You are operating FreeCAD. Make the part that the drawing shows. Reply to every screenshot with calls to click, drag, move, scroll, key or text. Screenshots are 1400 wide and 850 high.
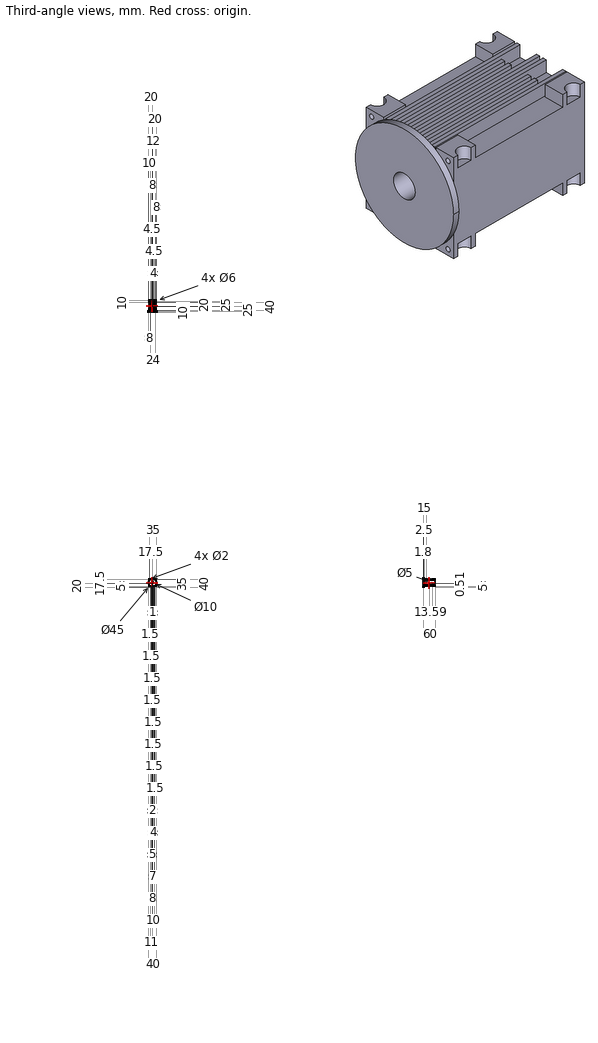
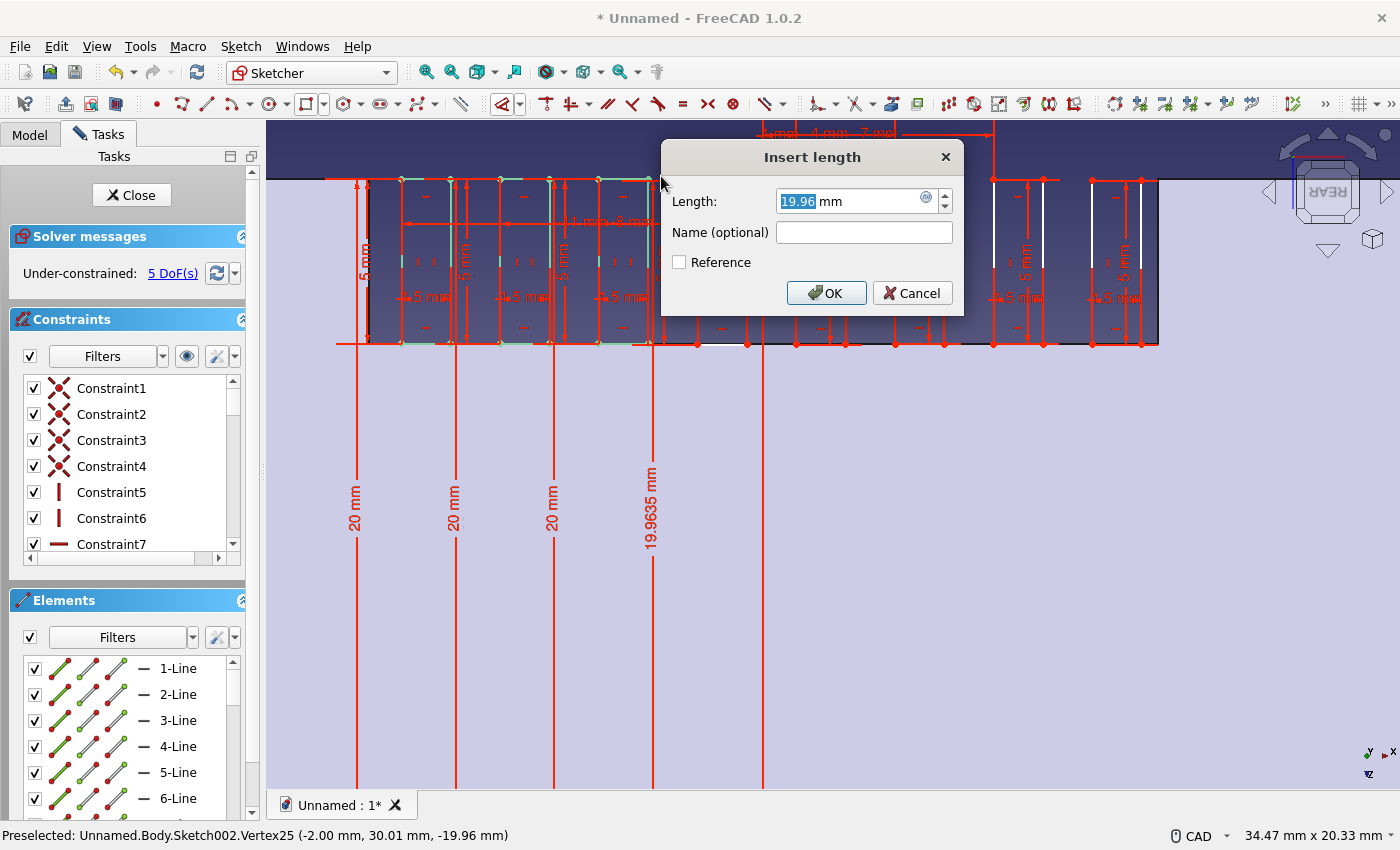
text(20)
key(Return)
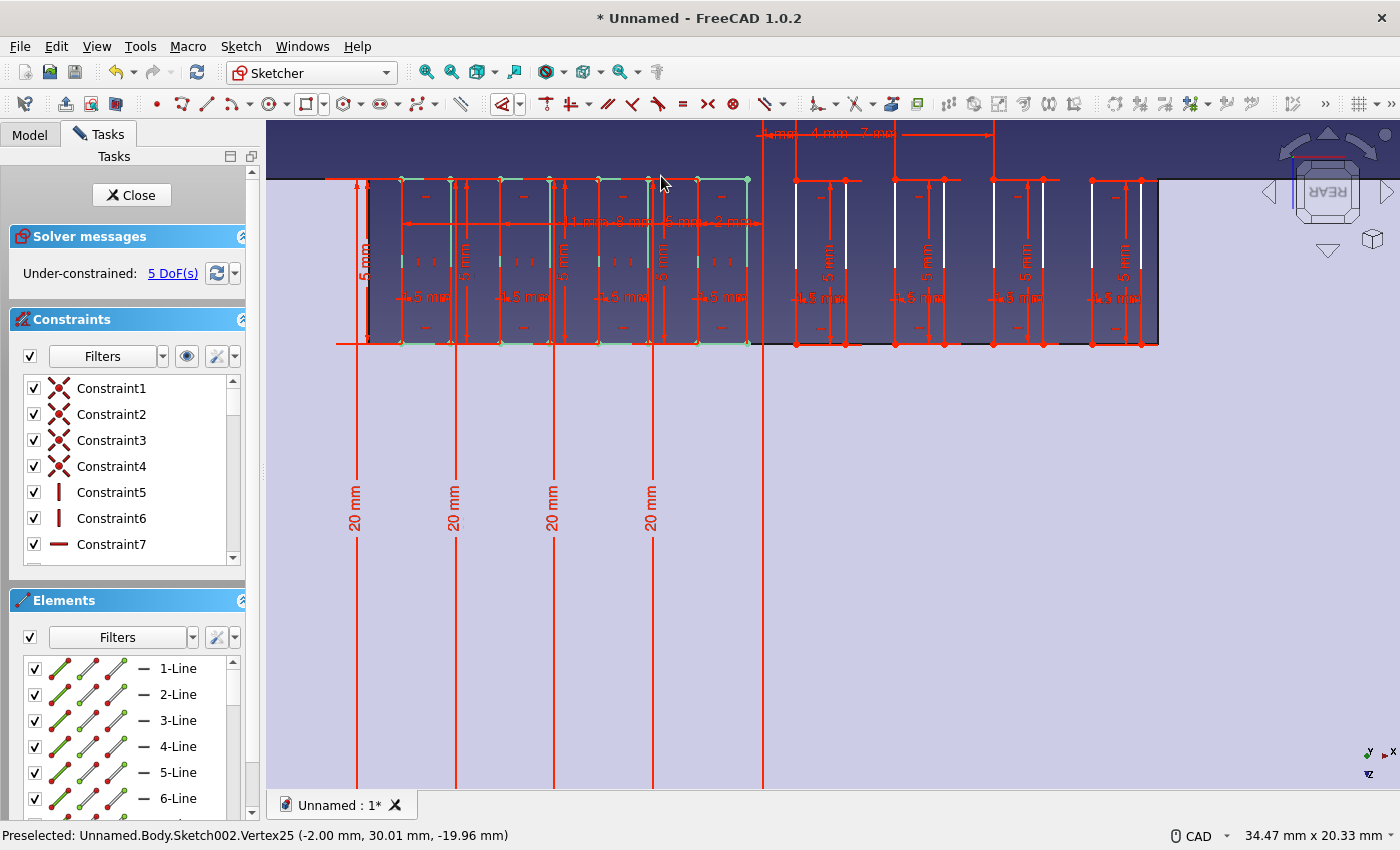
click(796, 181)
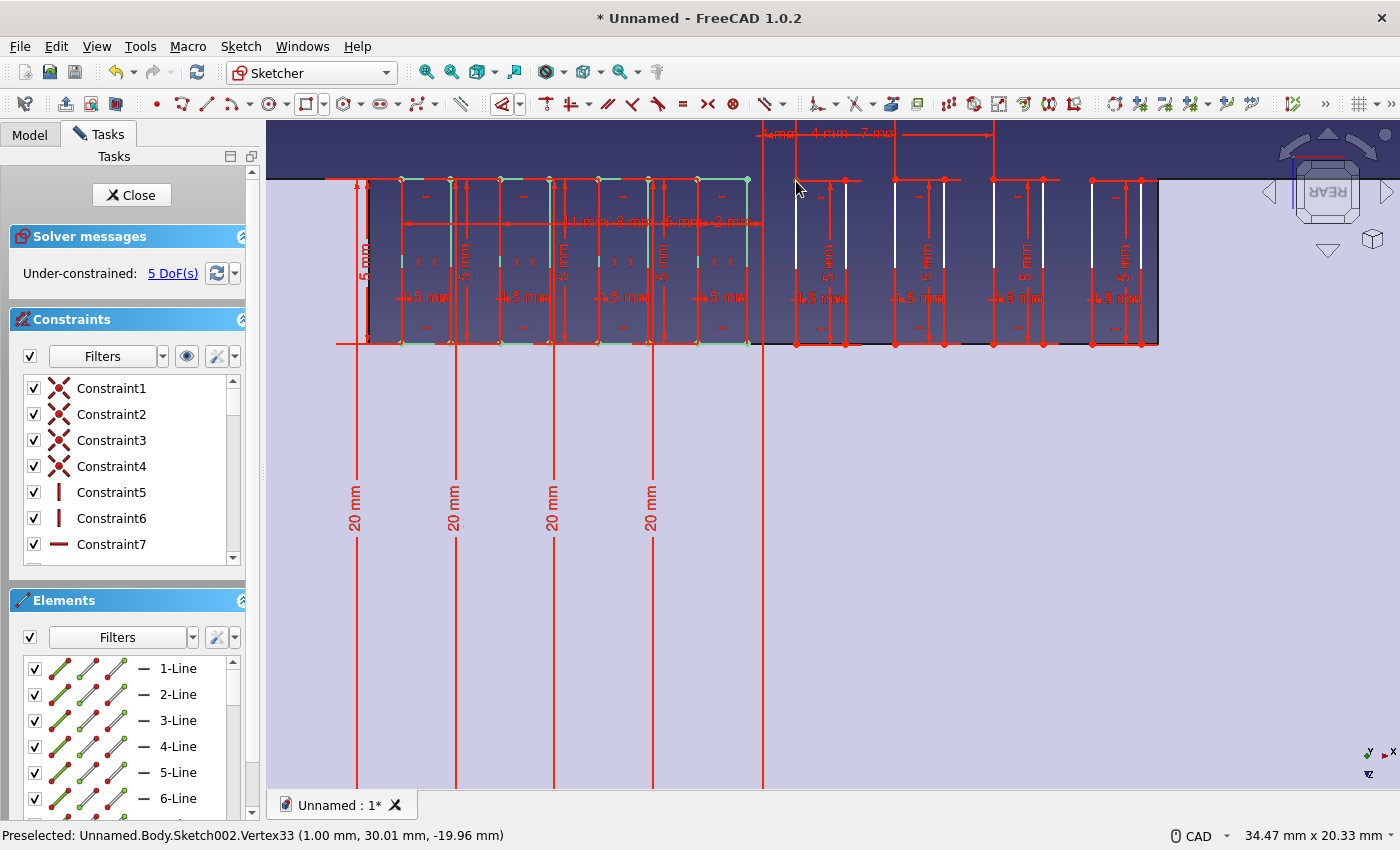
key(i)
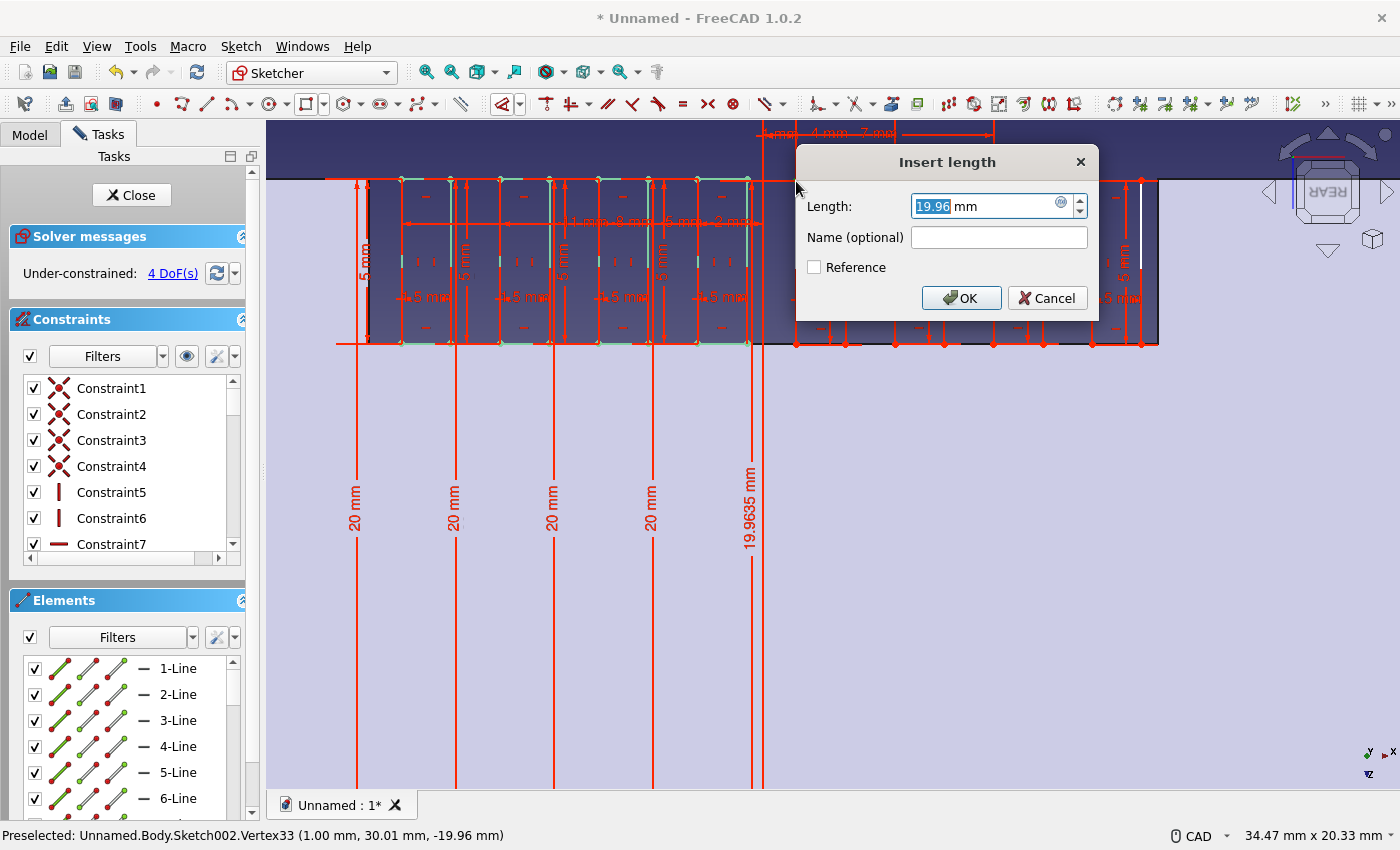
text(20)
key(Return)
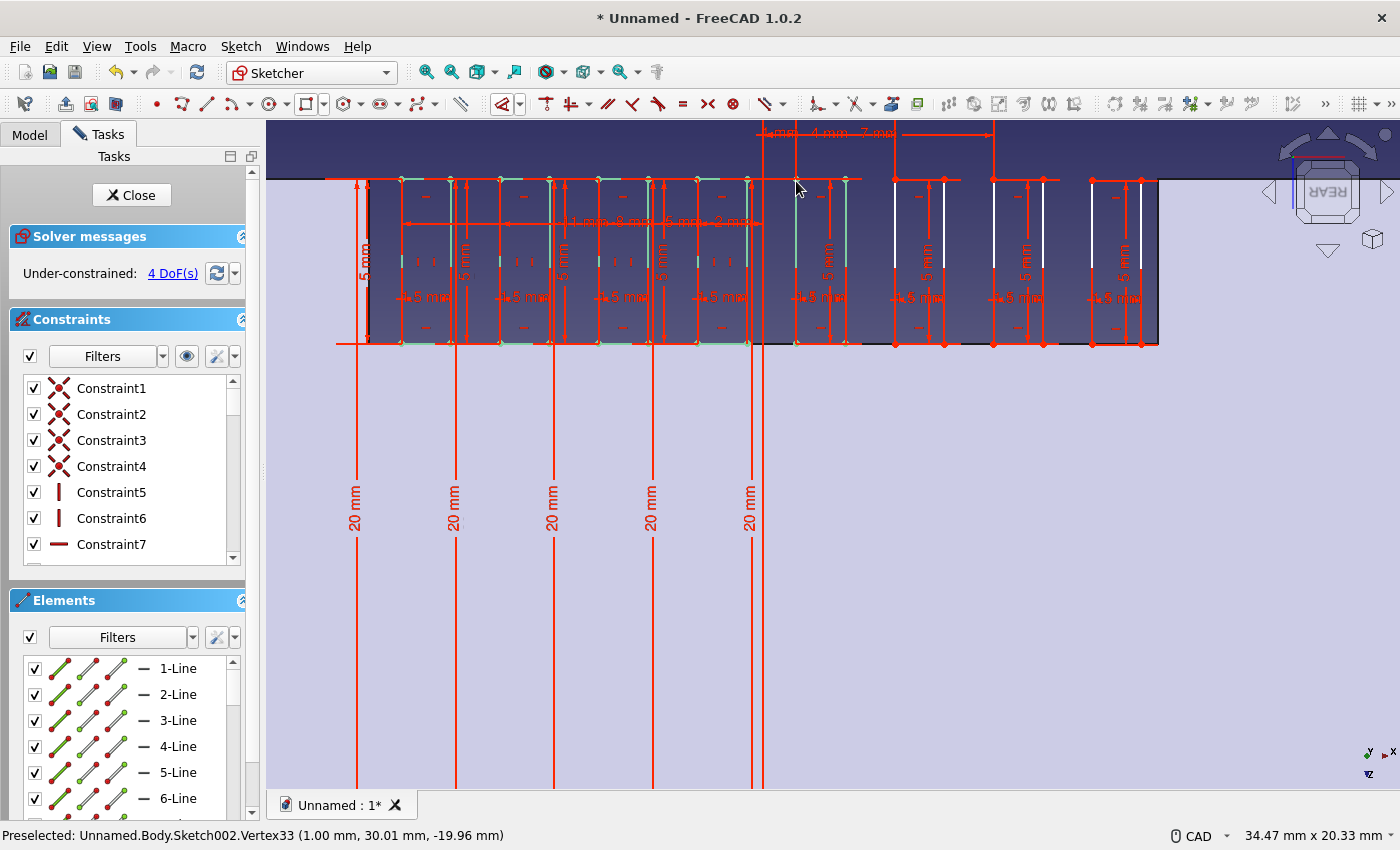
click(895, 180)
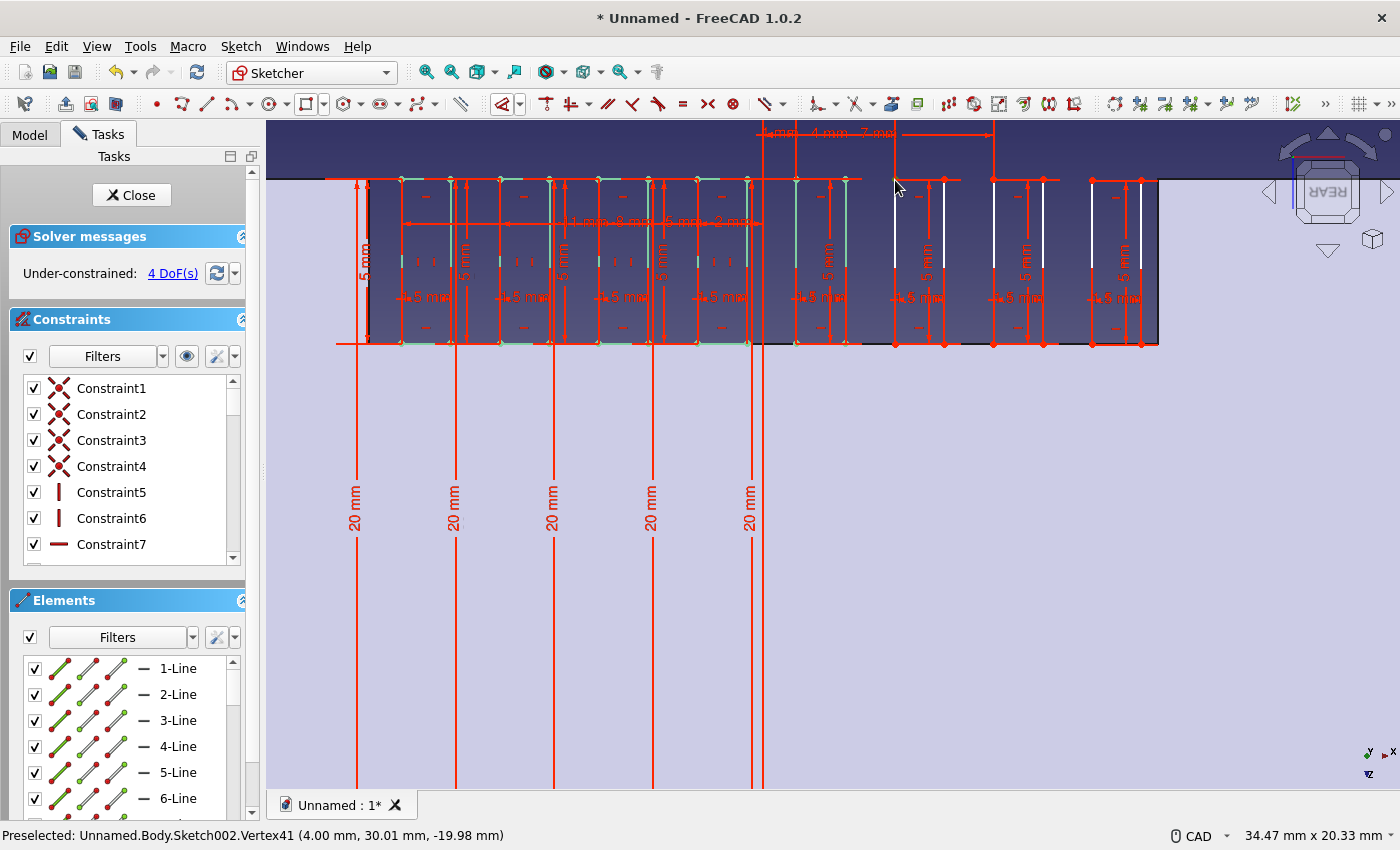
key(i)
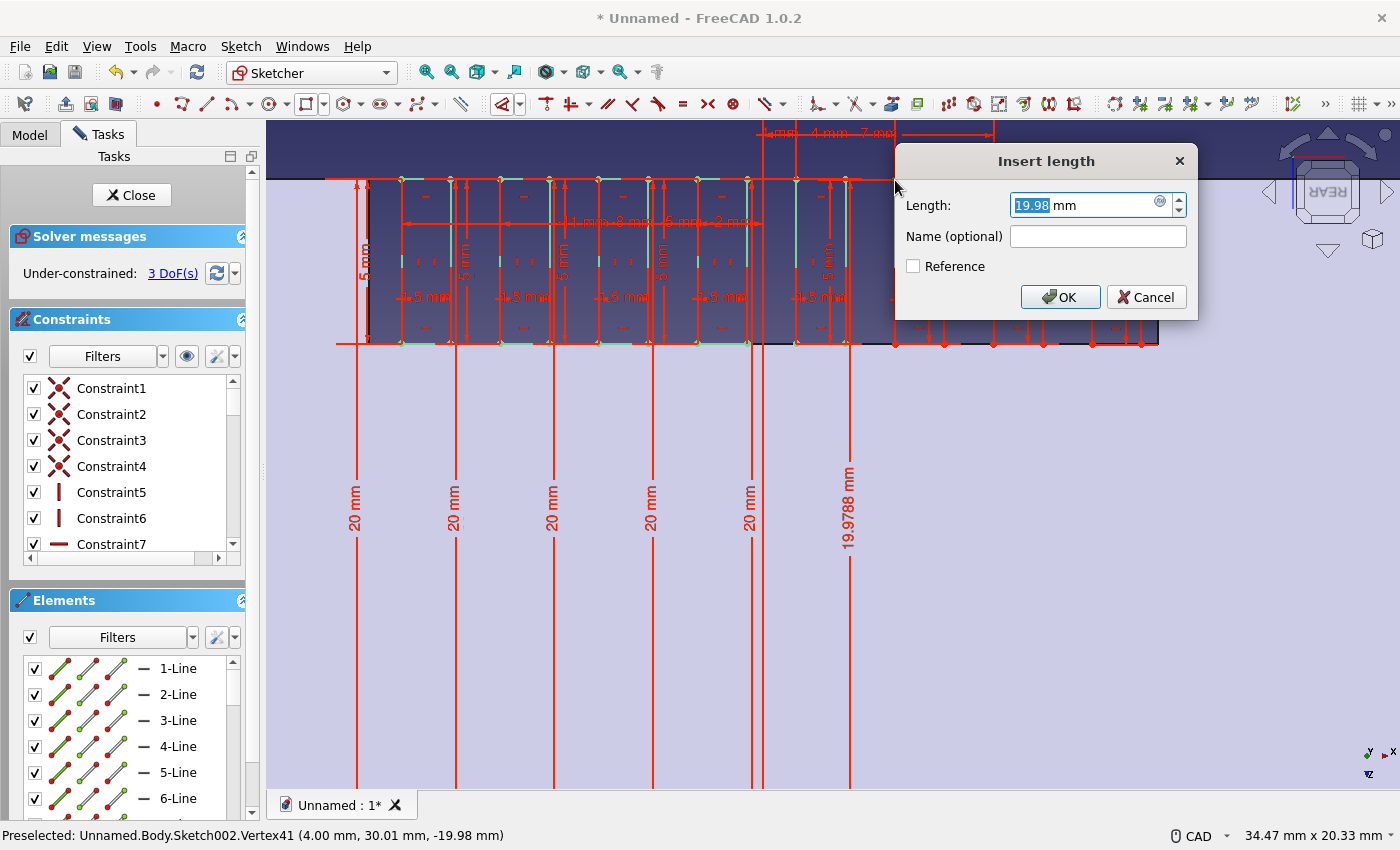
text(20)
key(Return)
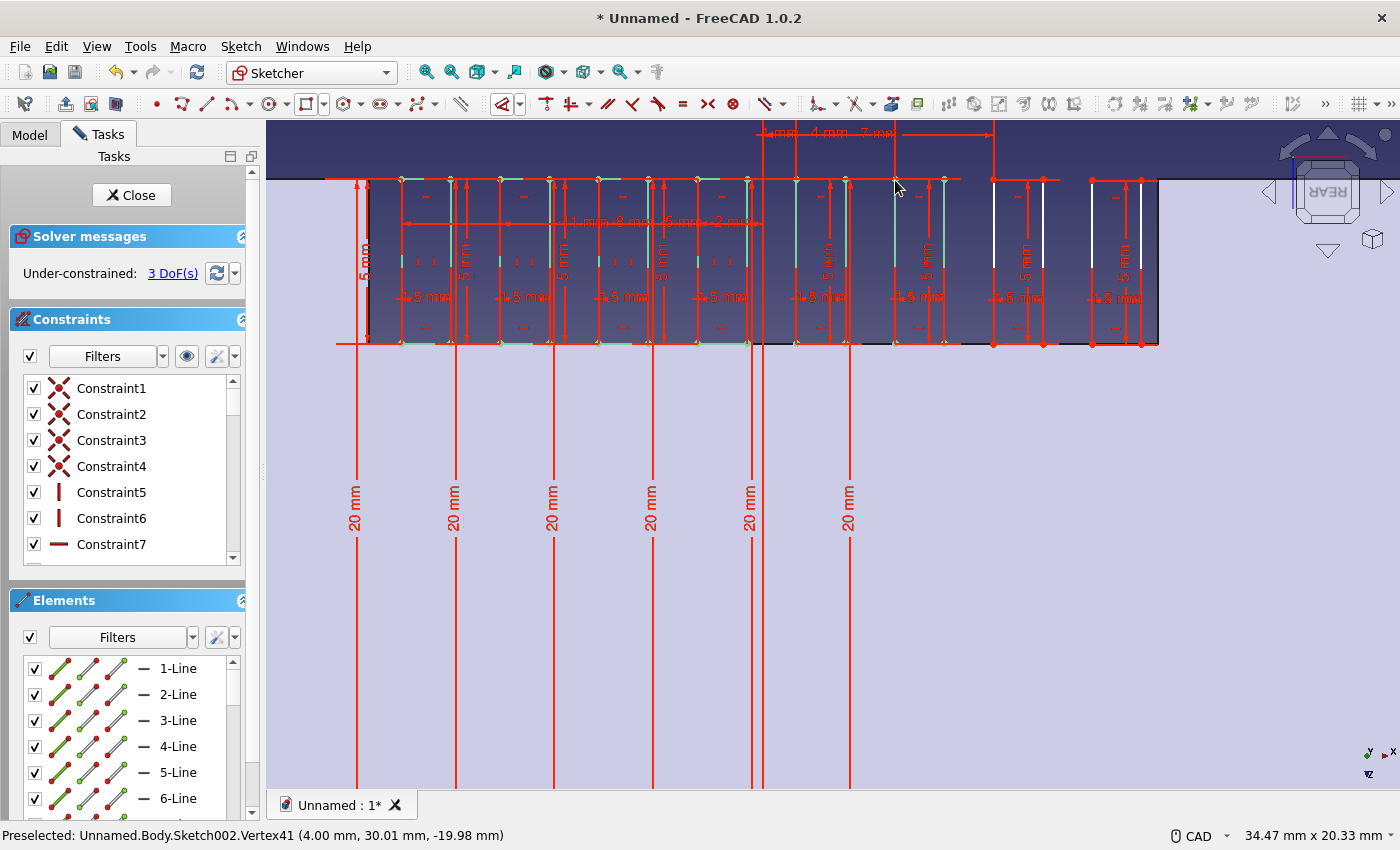
click(994, 180)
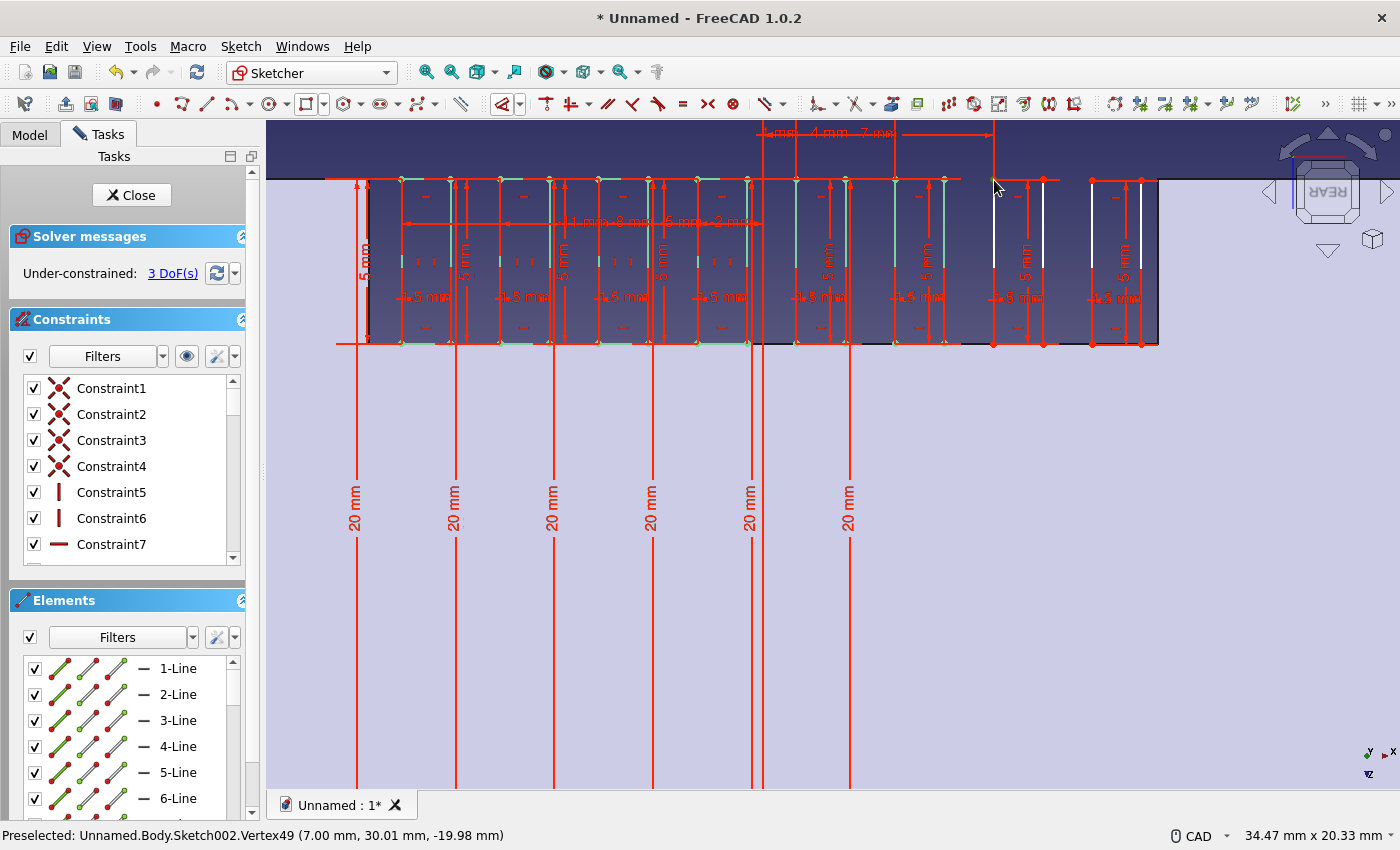
key(i)